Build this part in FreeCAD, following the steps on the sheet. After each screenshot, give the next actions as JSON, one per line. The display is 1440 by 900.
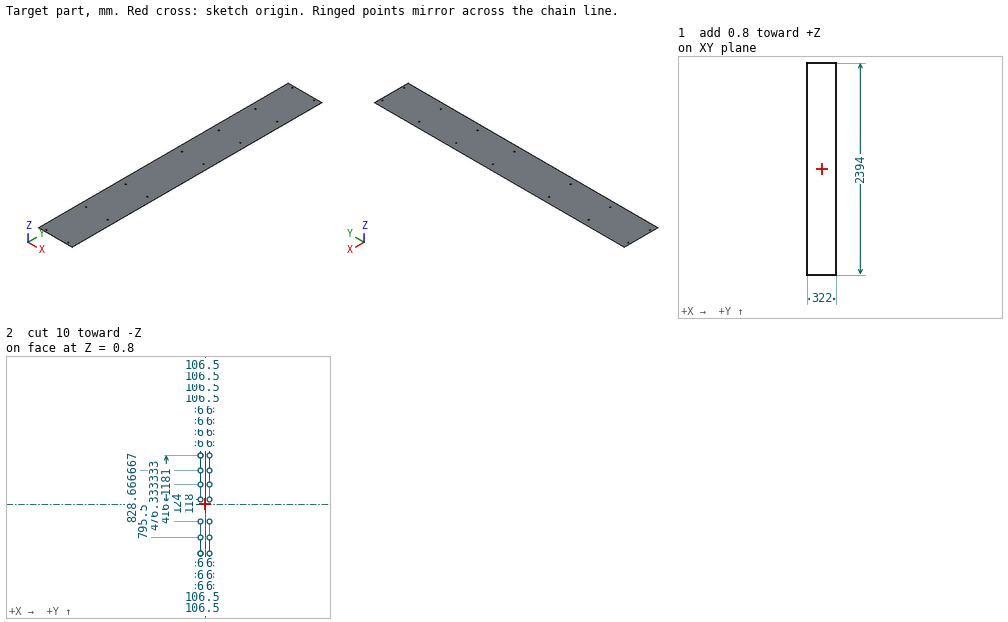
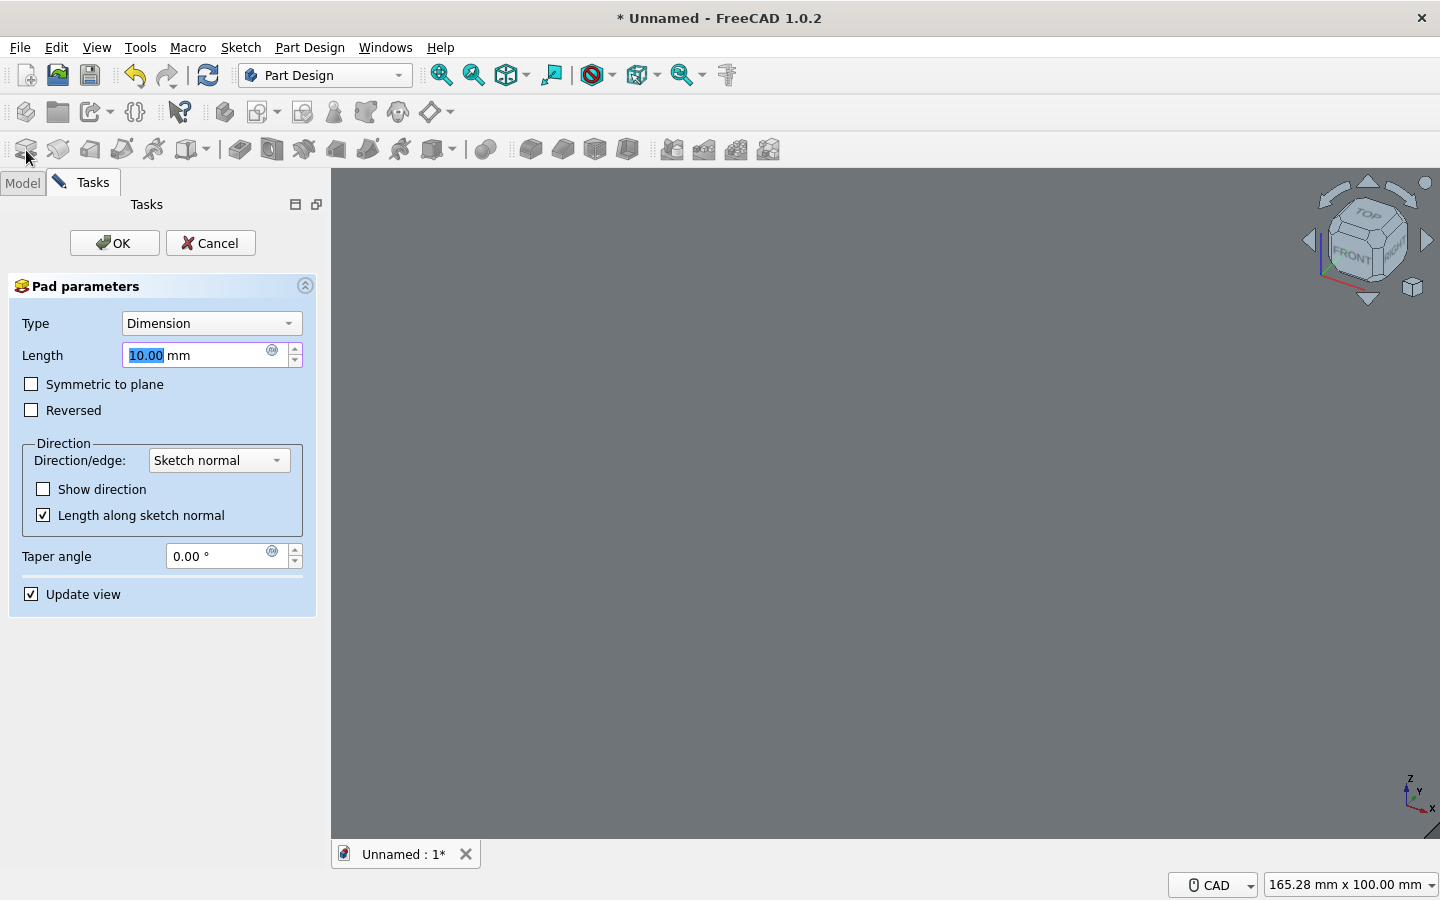
{"action": "type", "text": "0.8"}
{"action": "key", "text": "Tab"}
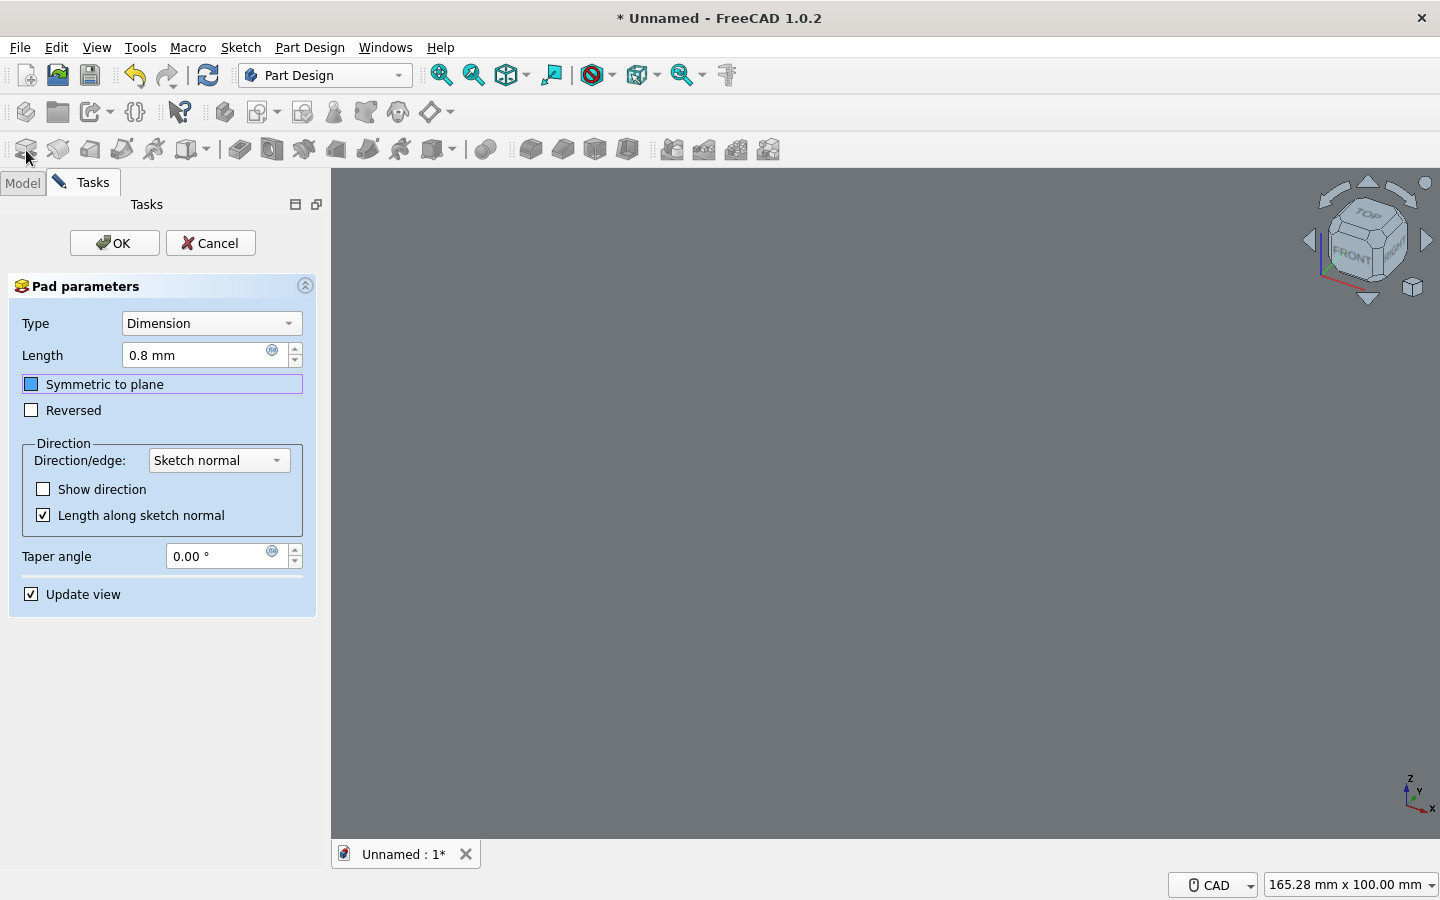
{"action": "left_click", "coordinate": [115, 243]}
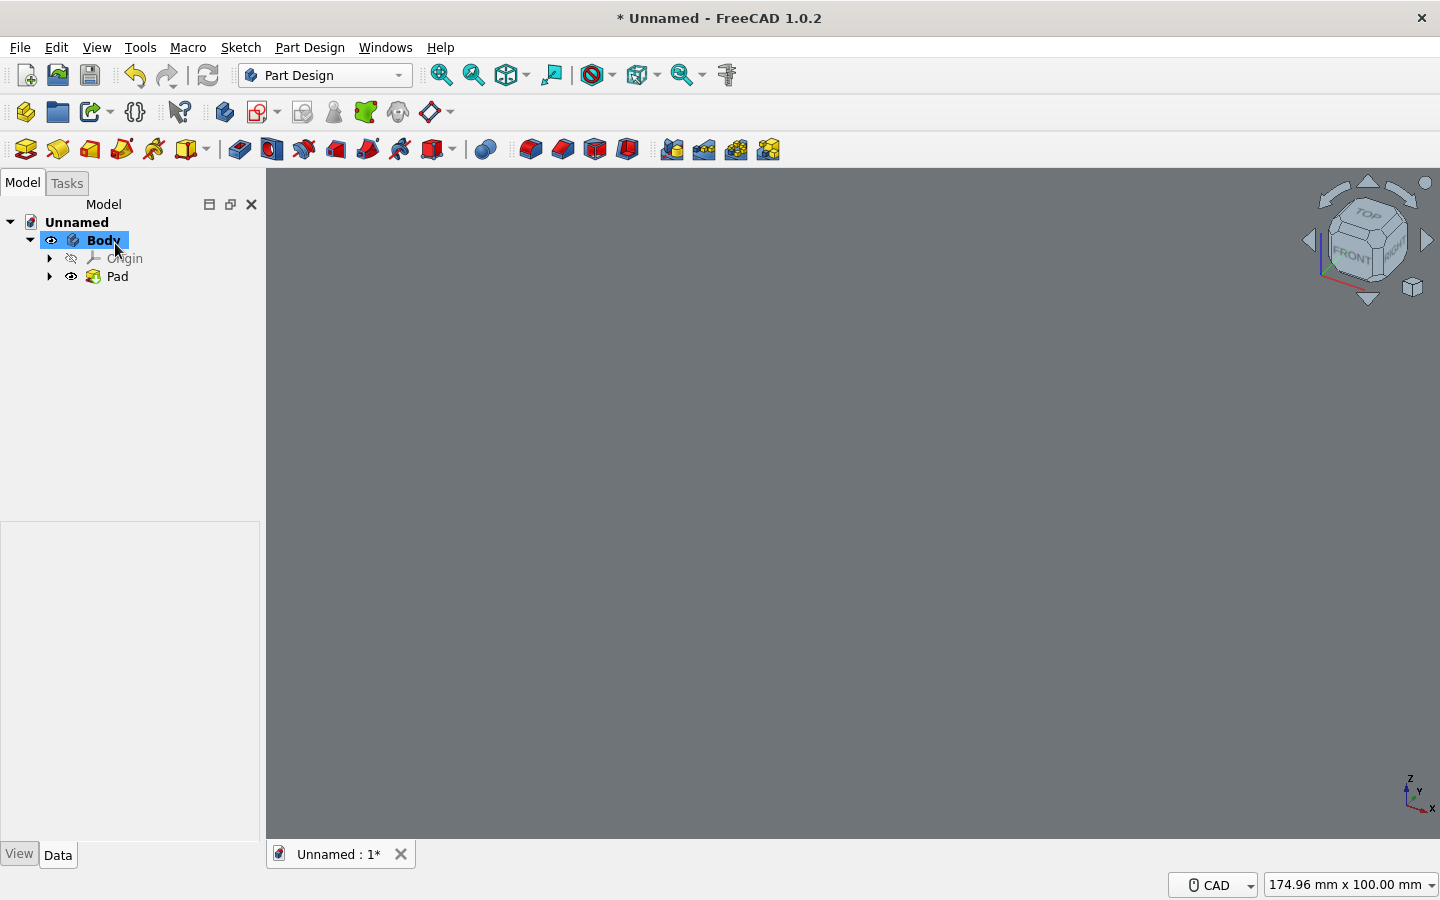
{"action": "key", "text": "v f"}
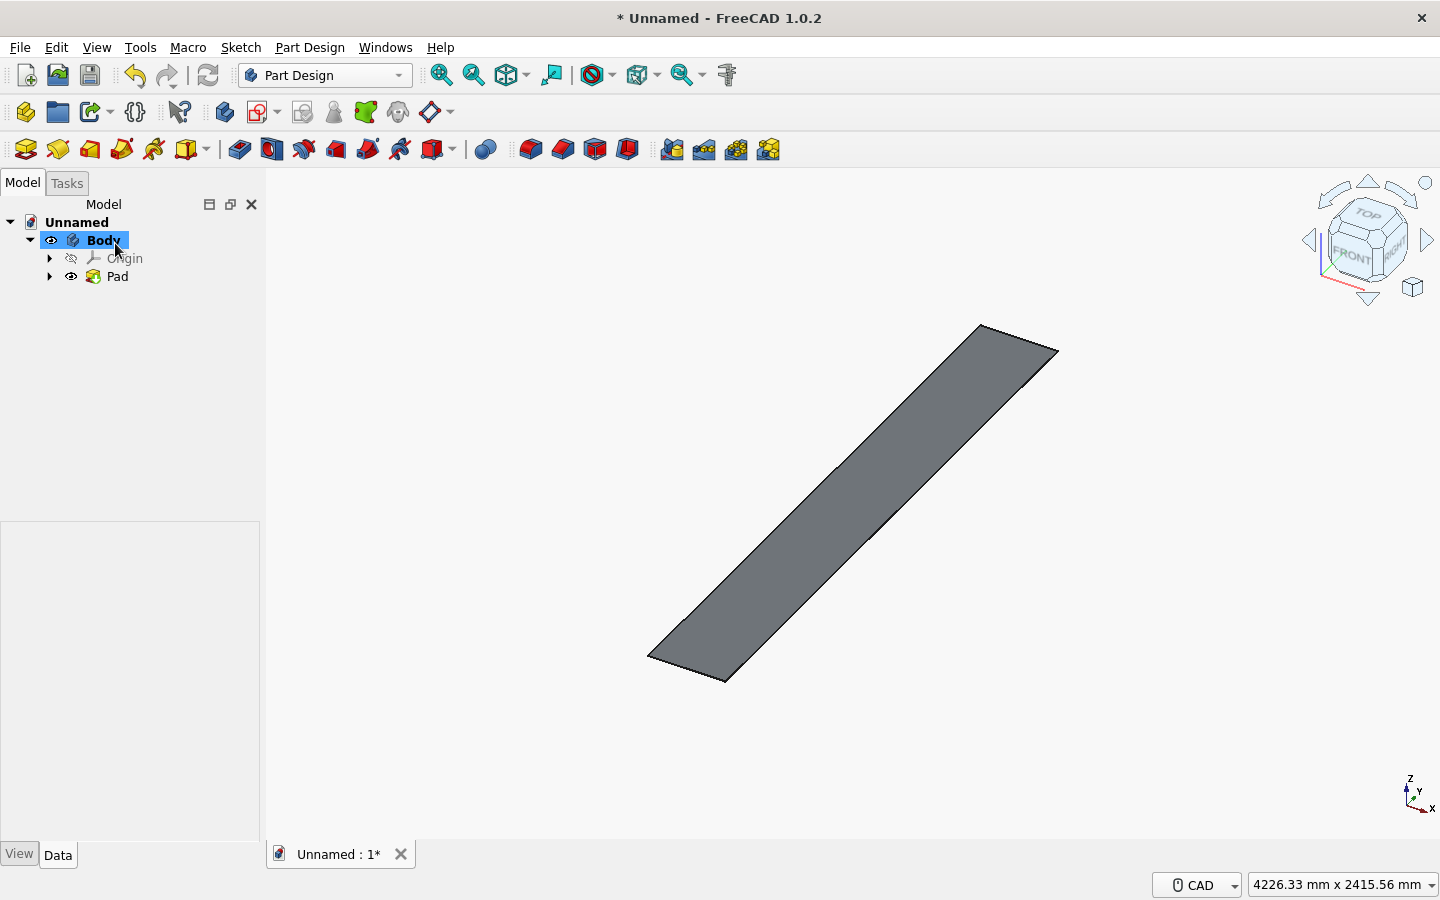
{"action": "left_click", "coordinate": [996, 361]}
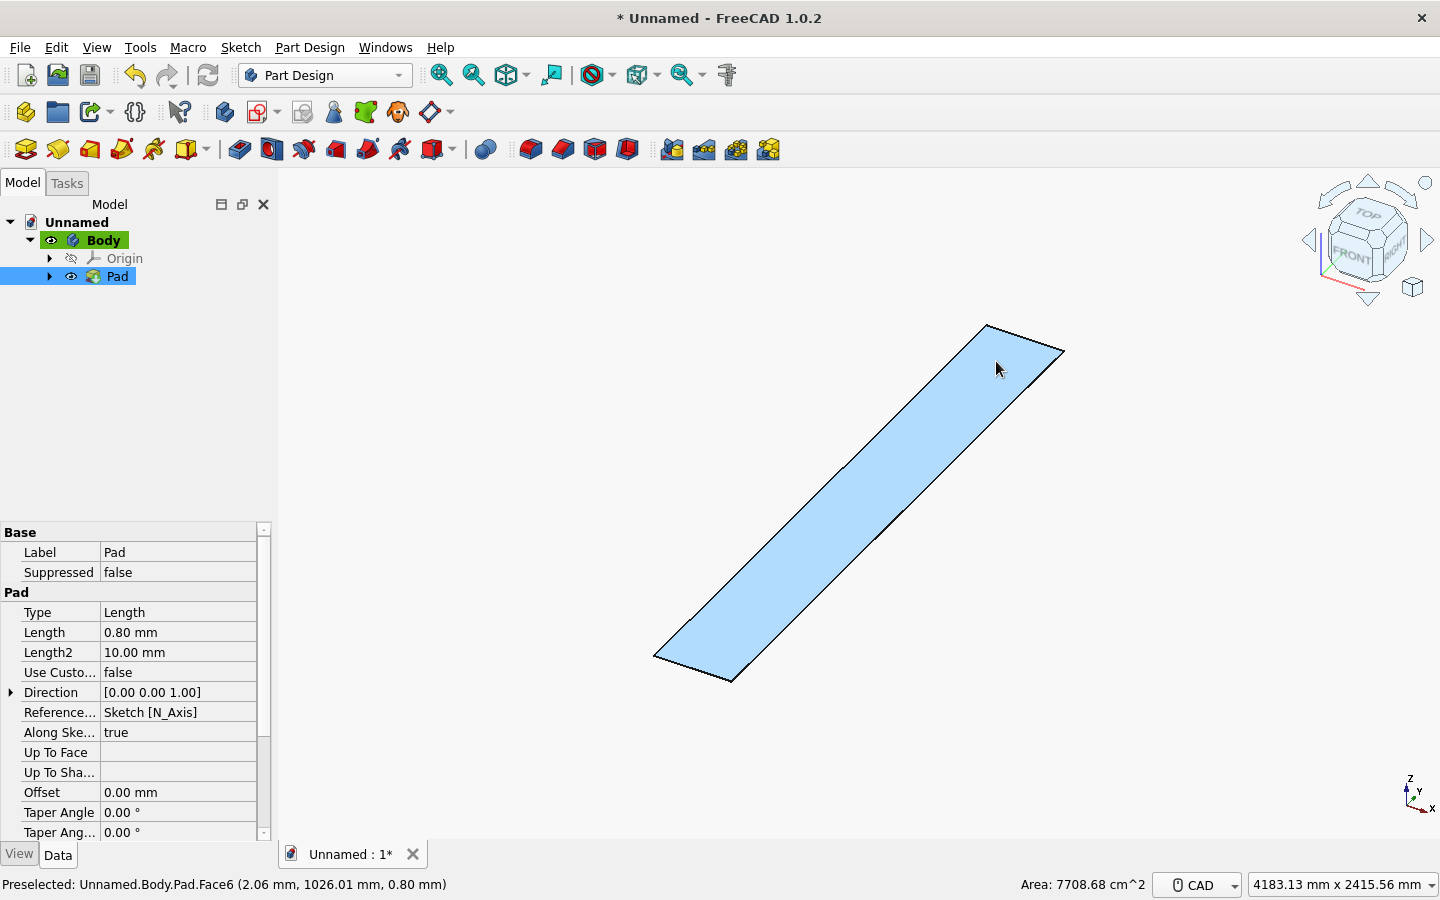
{"action": "left_click", "coordinate": [258, 112]}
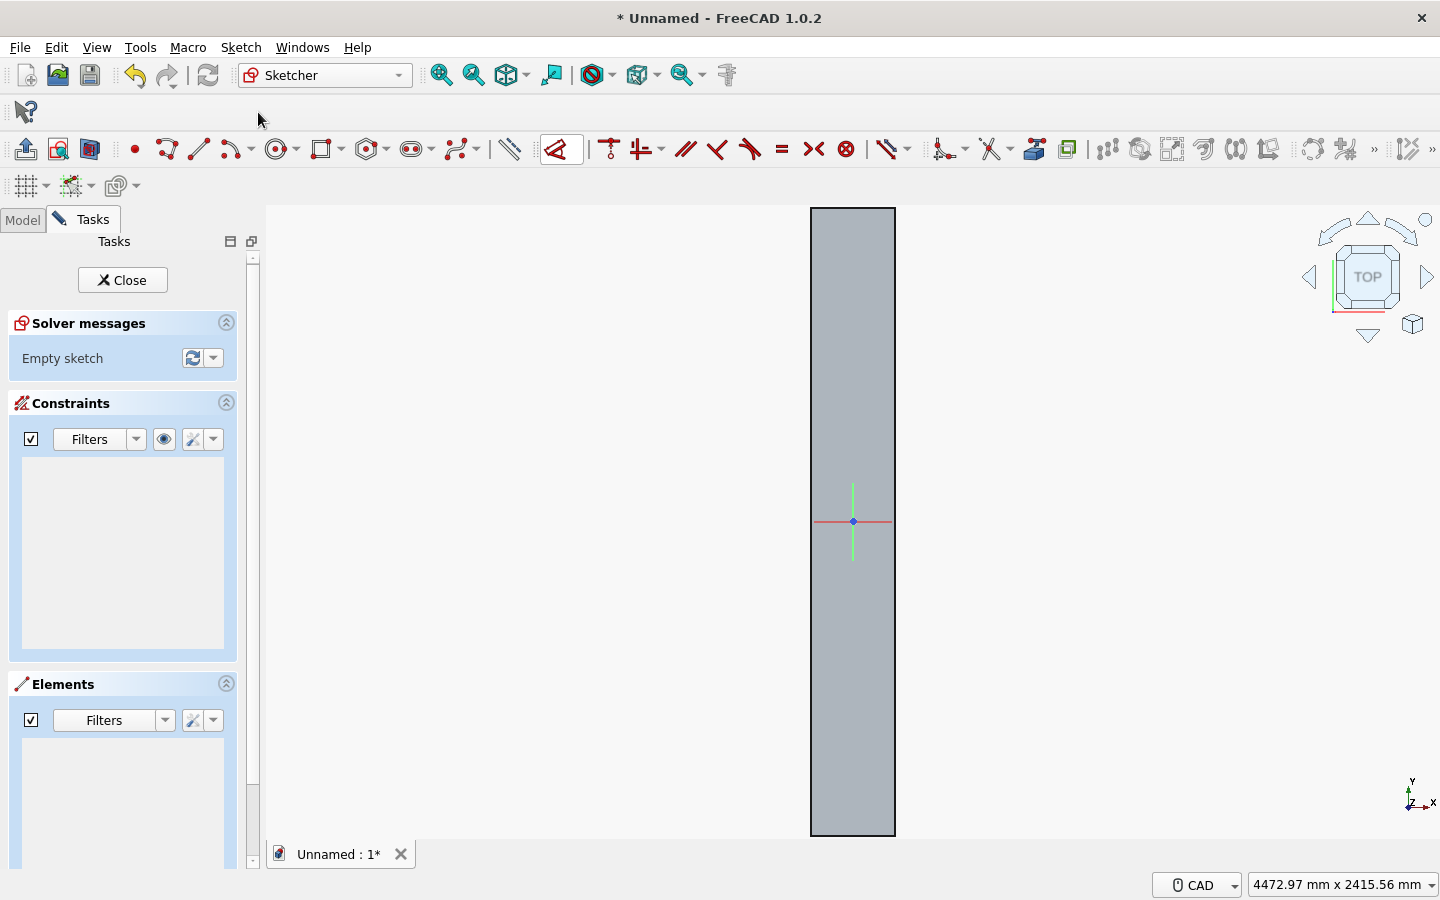
{"action": "scroll", "coordinate": [645, 522], "scroll_direction": "down", "scroll_amount": 2}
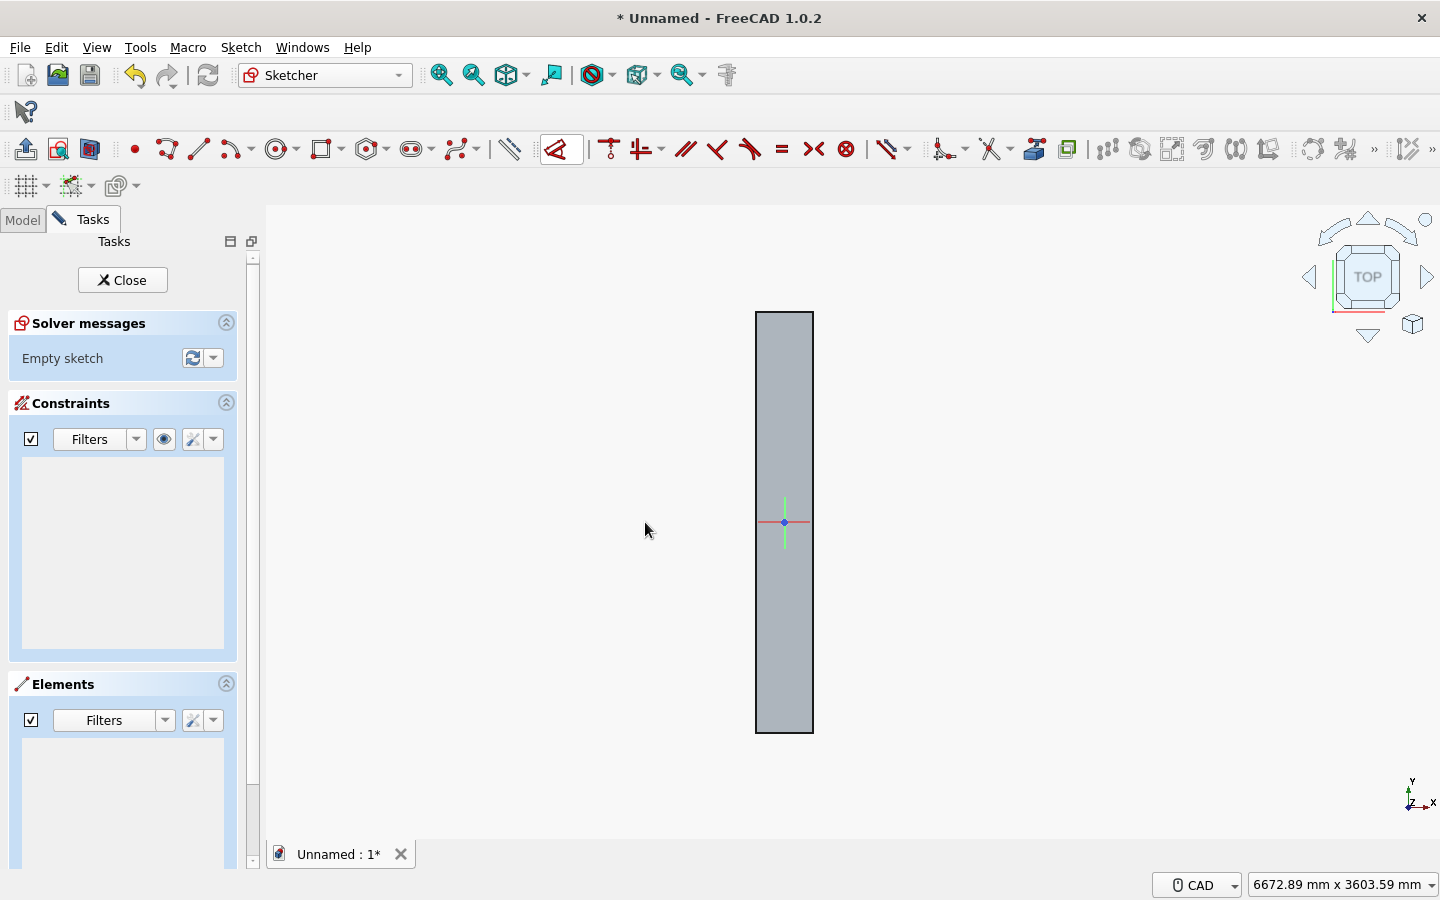
{"action": "key", "text": "g s"}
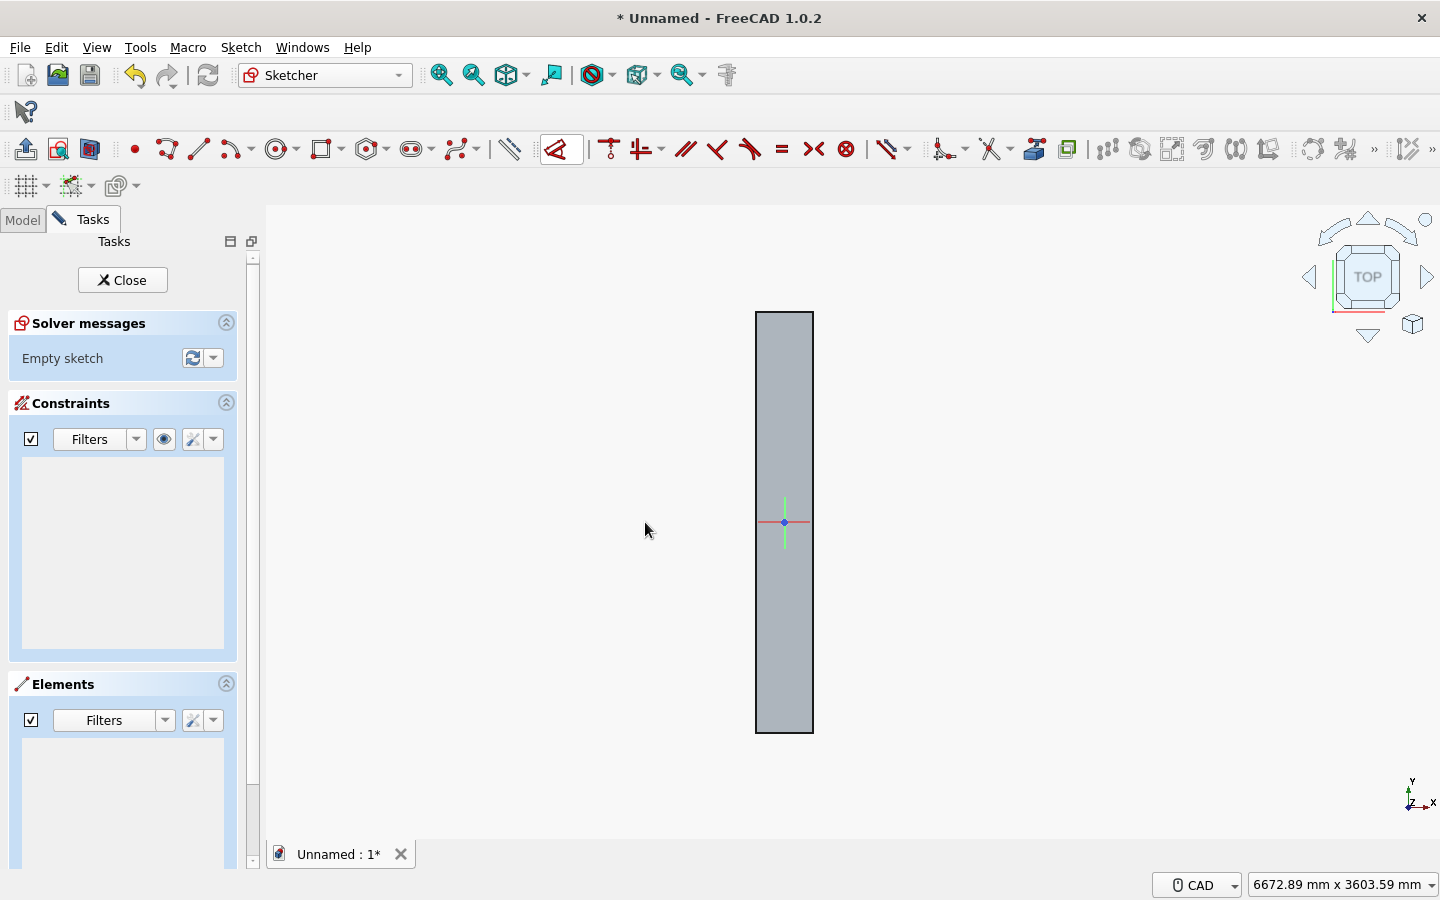
{"action": "scroll", "coordinate": [766, 501], "scroll_direction": "up", "scroll_amount": 19}